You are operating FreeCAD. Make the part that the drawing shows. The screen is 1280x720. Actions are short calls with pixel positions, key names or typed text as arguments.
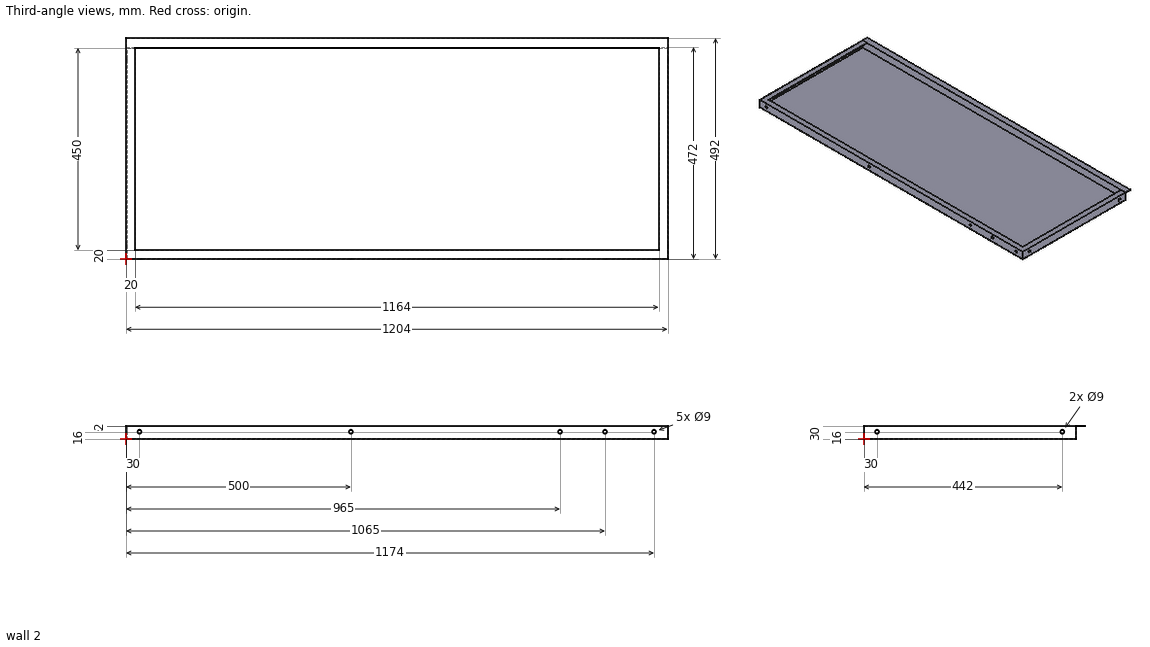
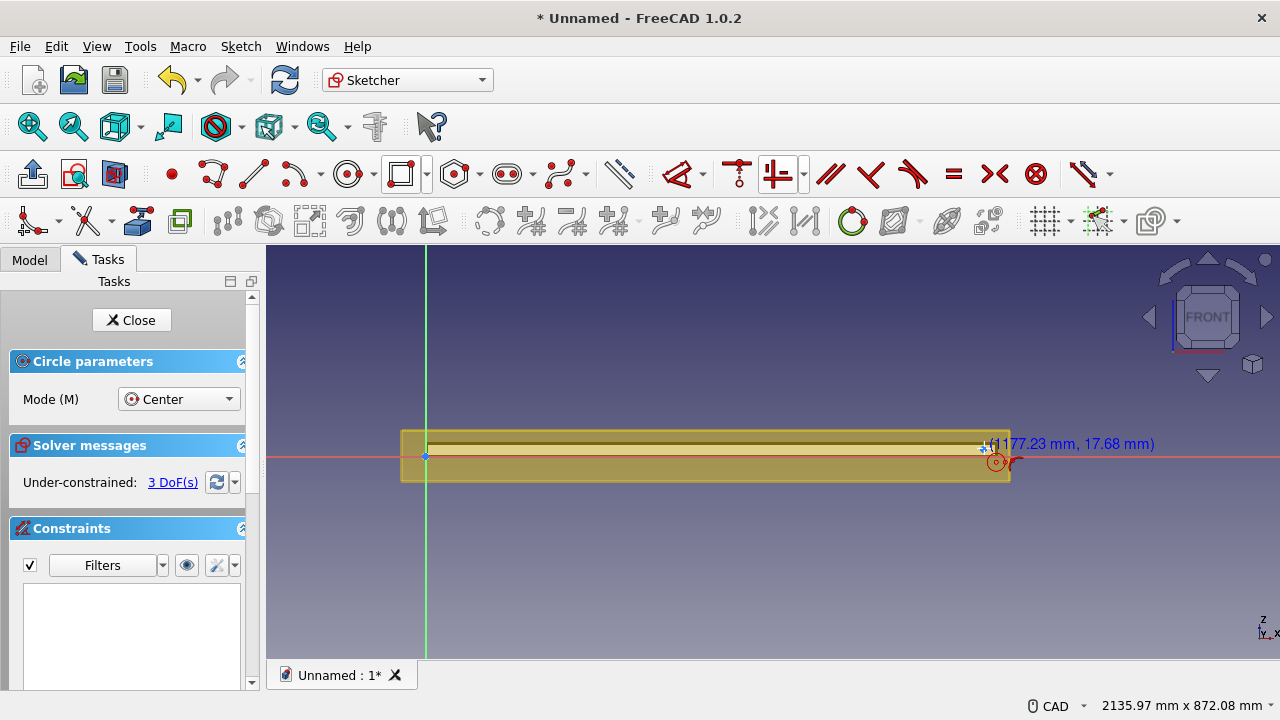
scroll(440, 449, up, 12)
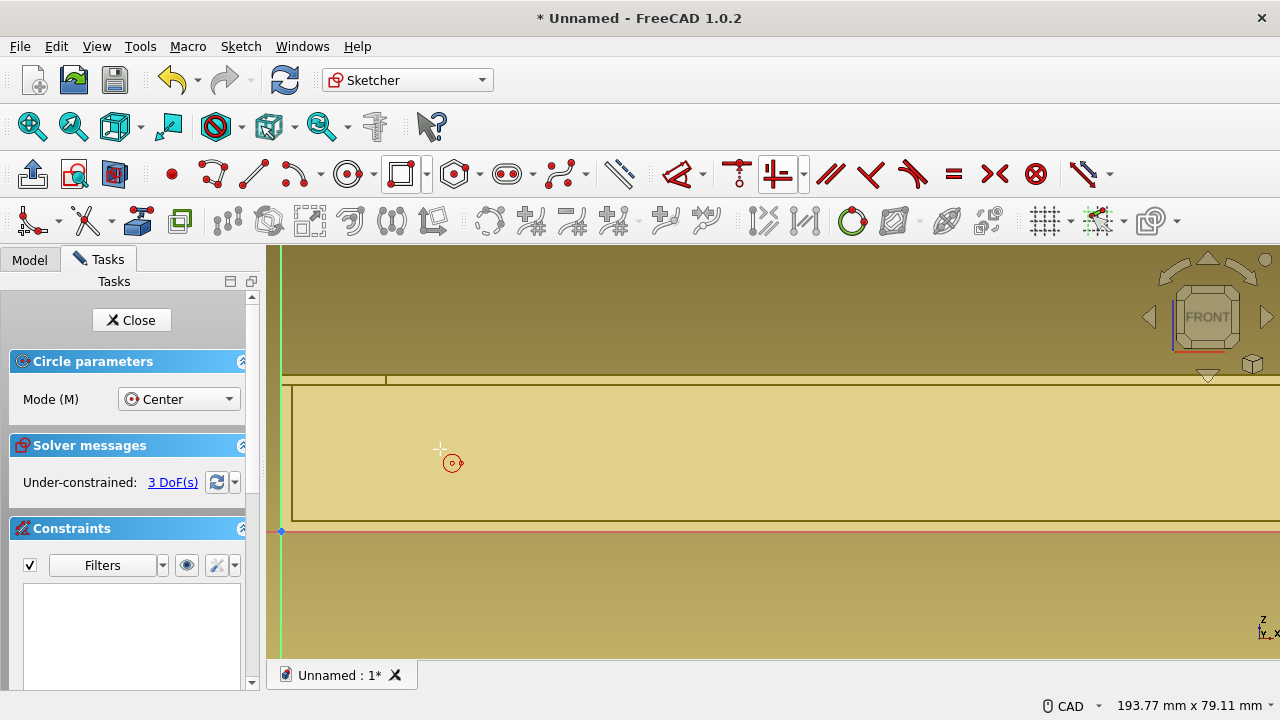
scroll(439, 449, down, 12)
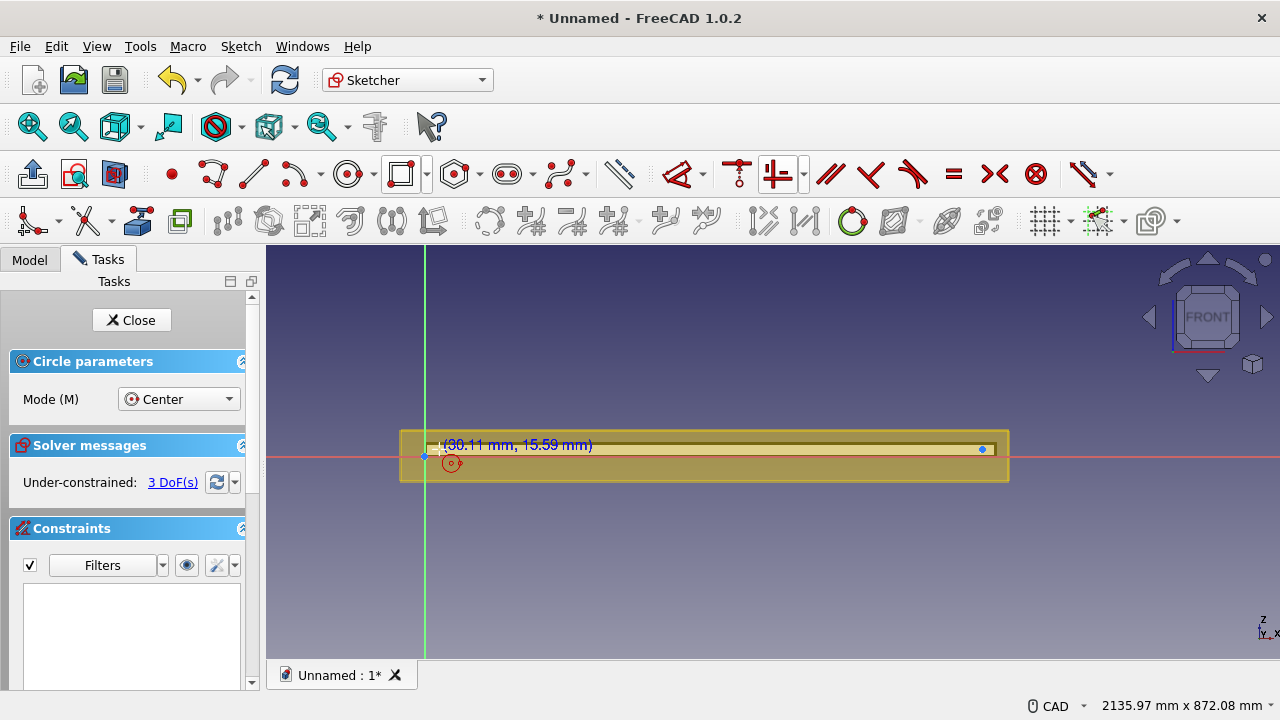
scroll(439, 449, up, 4)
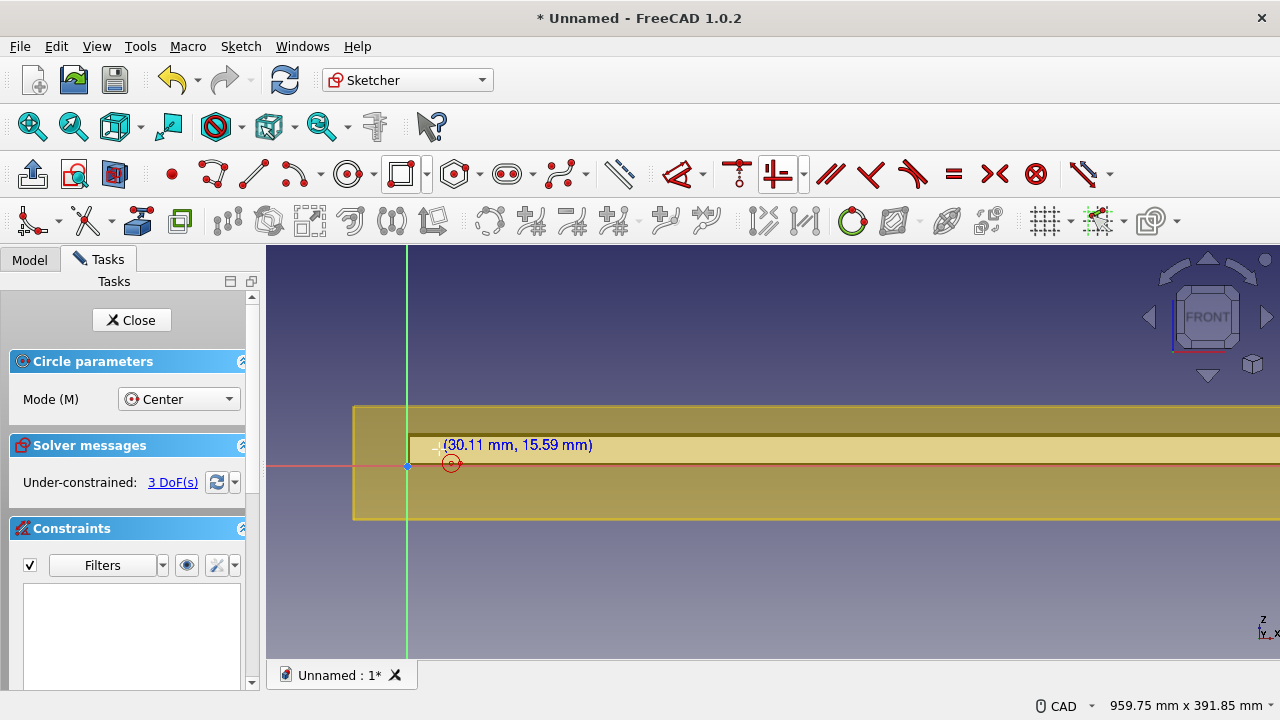
click(439, 449)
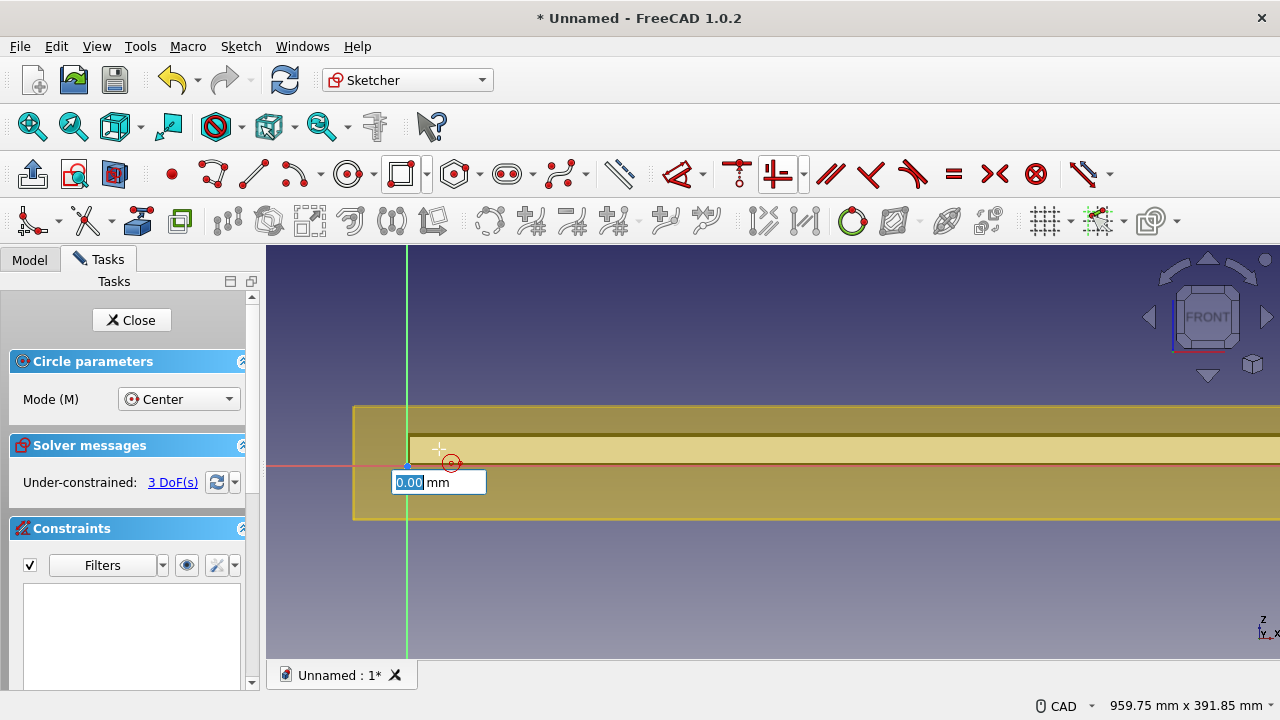
scroll(442, 446, up, 7)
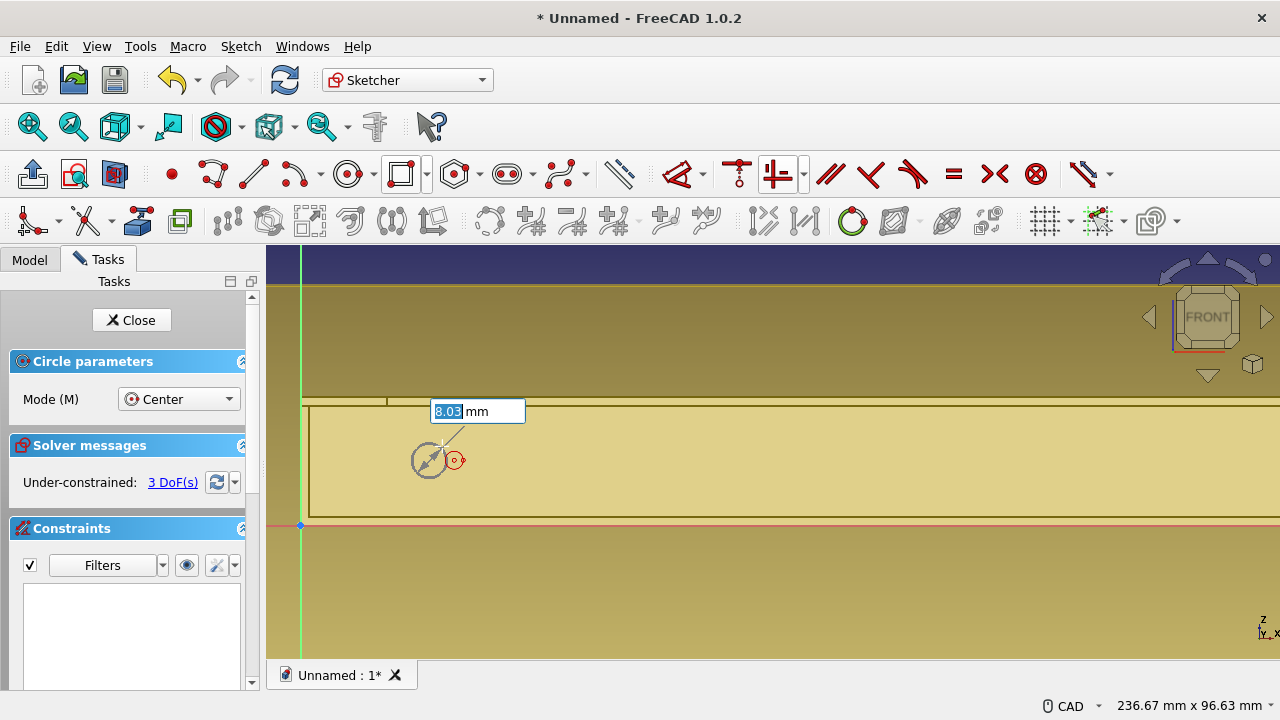
click(443, 444)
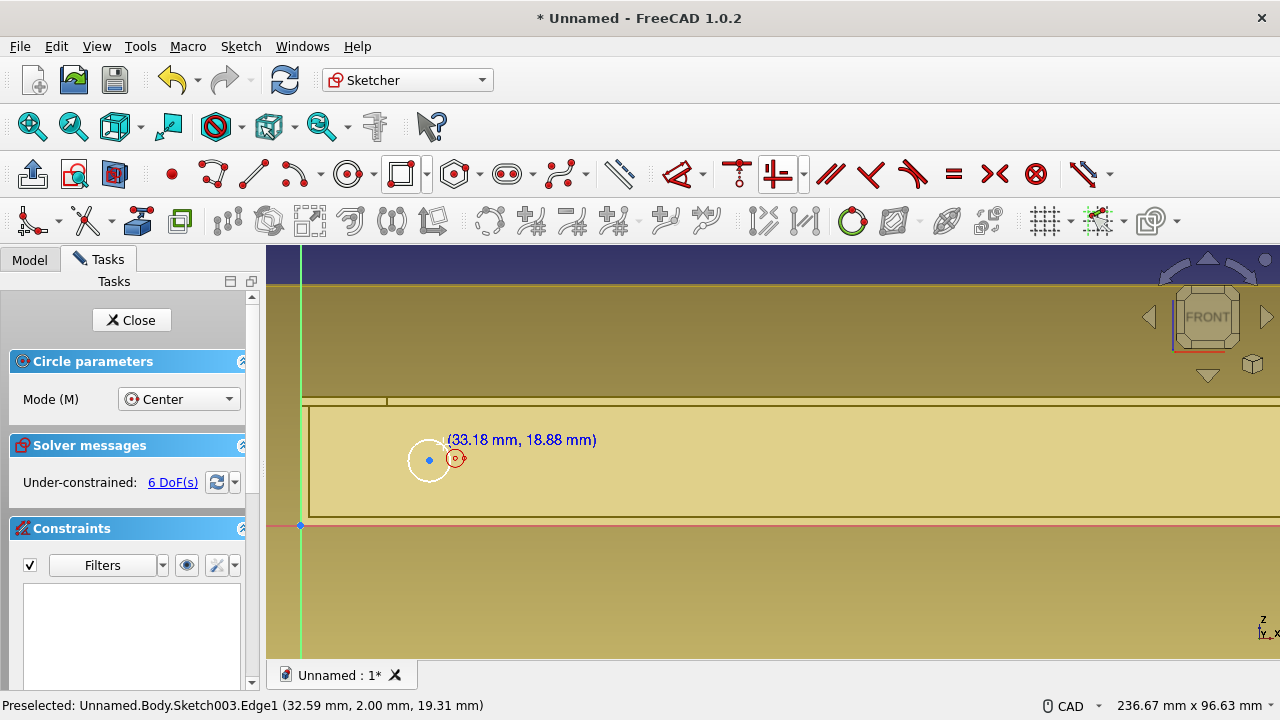
scroll(440, 448, down, 11)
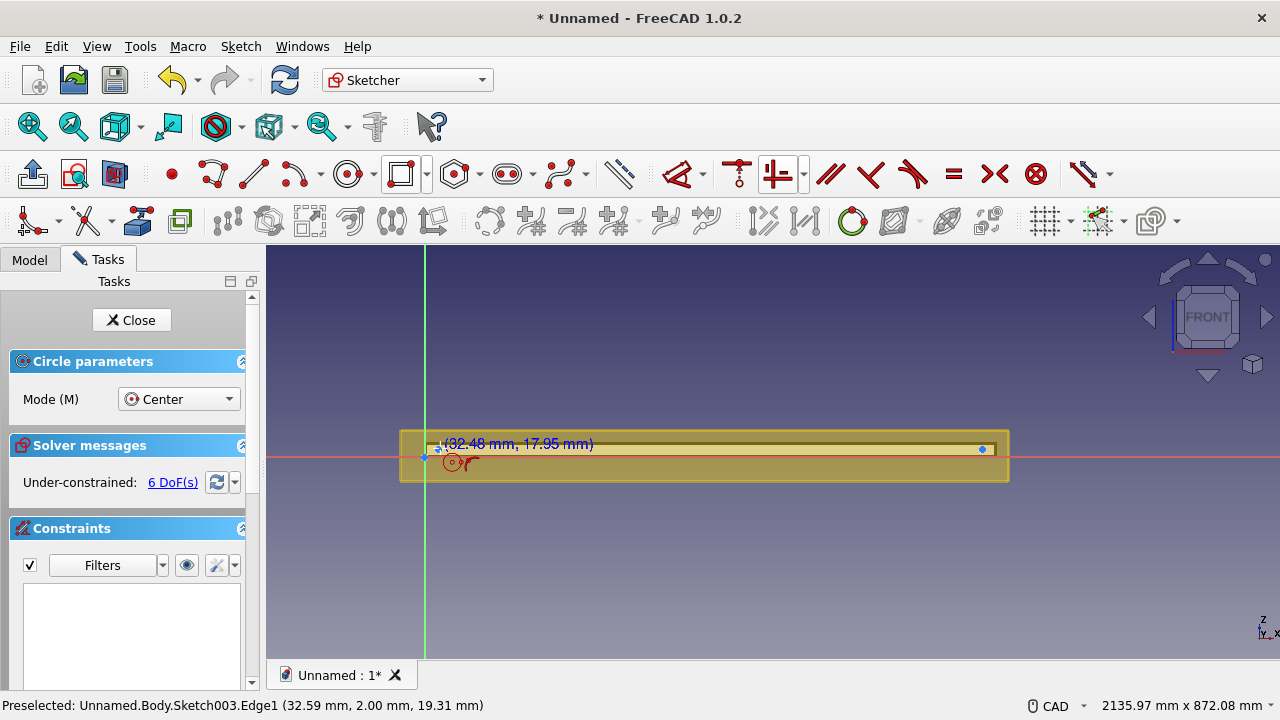
scroll(930, 449, up, 12)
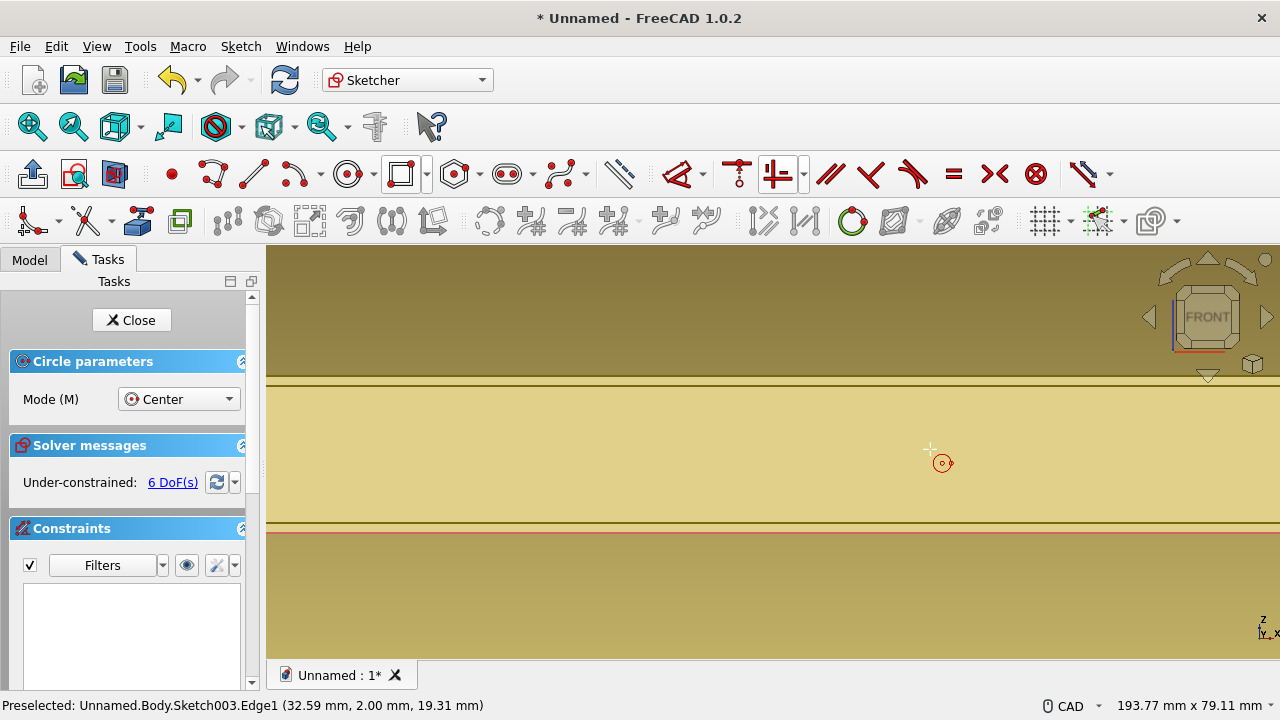
scroll(931, 449, down, 12)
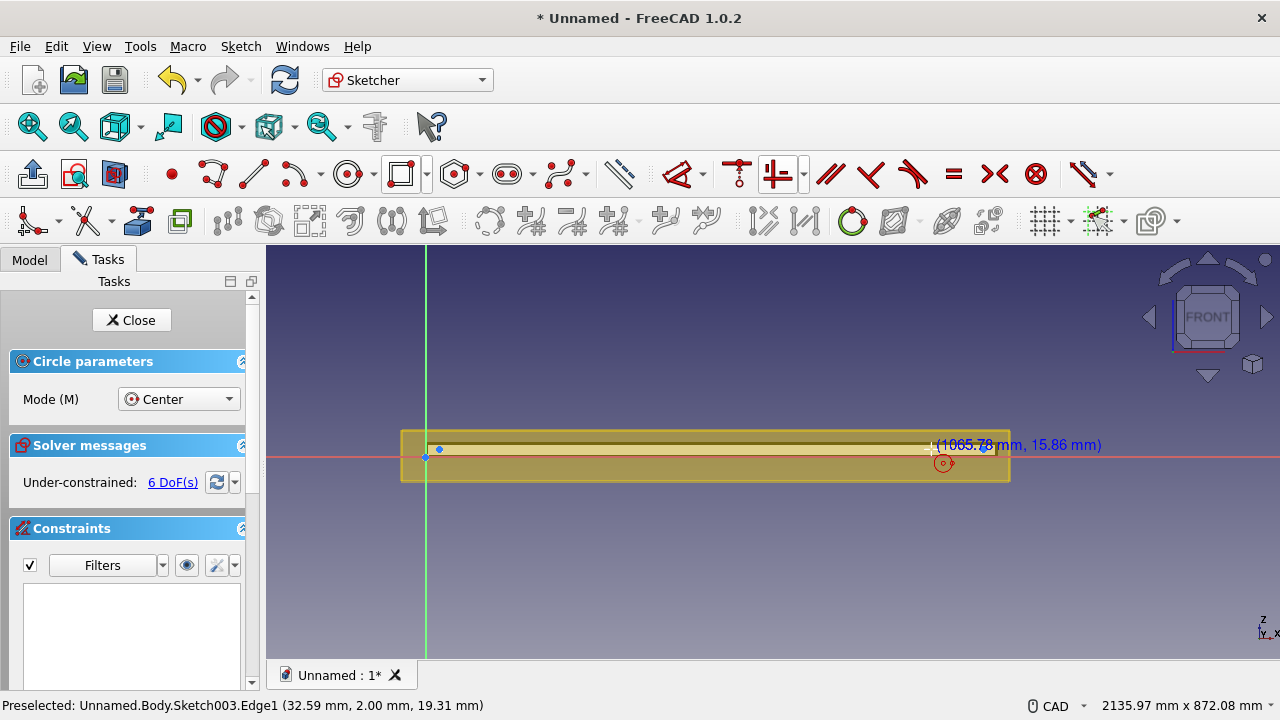
scroll(931, 449, up, 4)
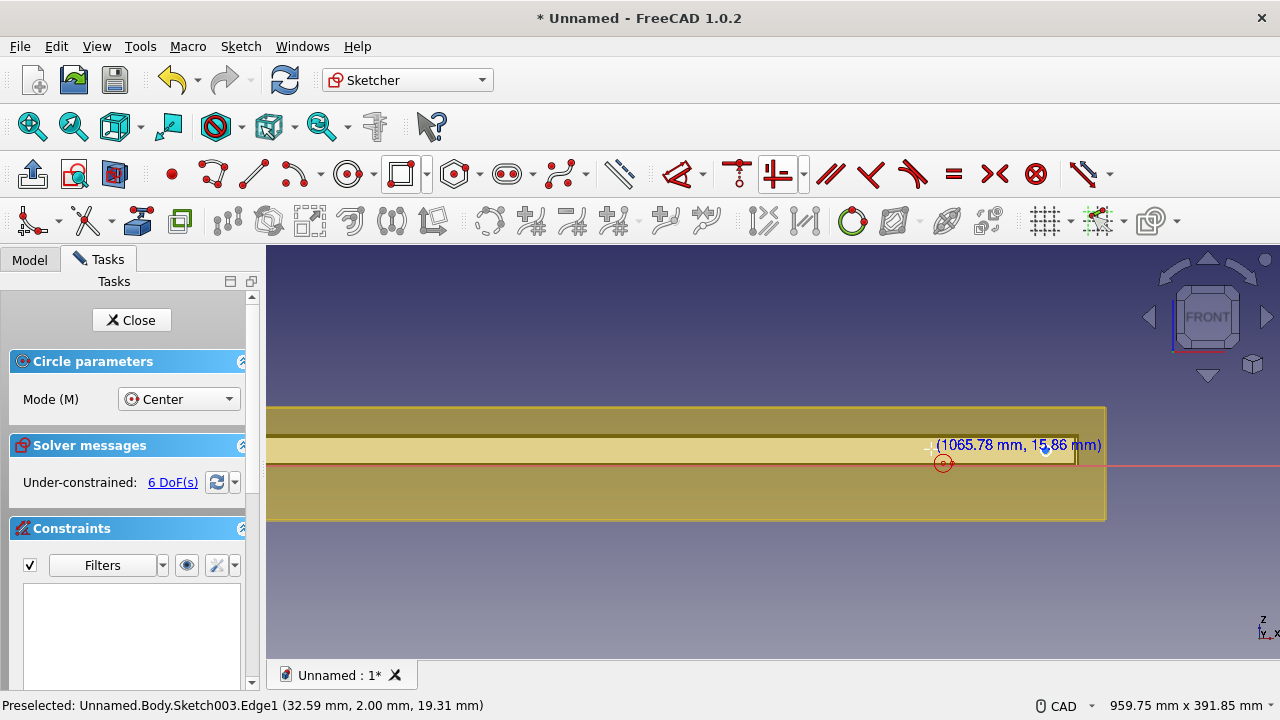
click(931, 449)